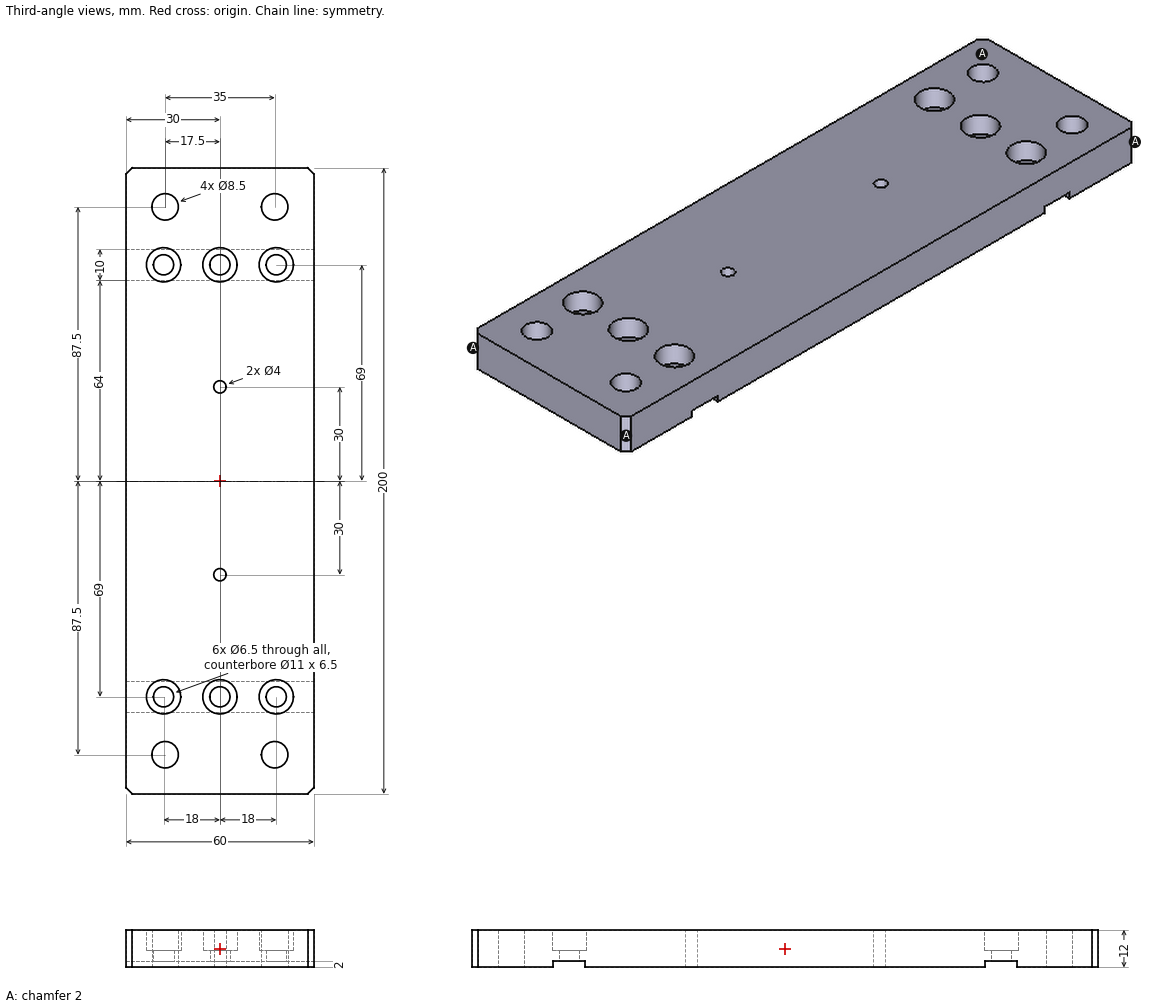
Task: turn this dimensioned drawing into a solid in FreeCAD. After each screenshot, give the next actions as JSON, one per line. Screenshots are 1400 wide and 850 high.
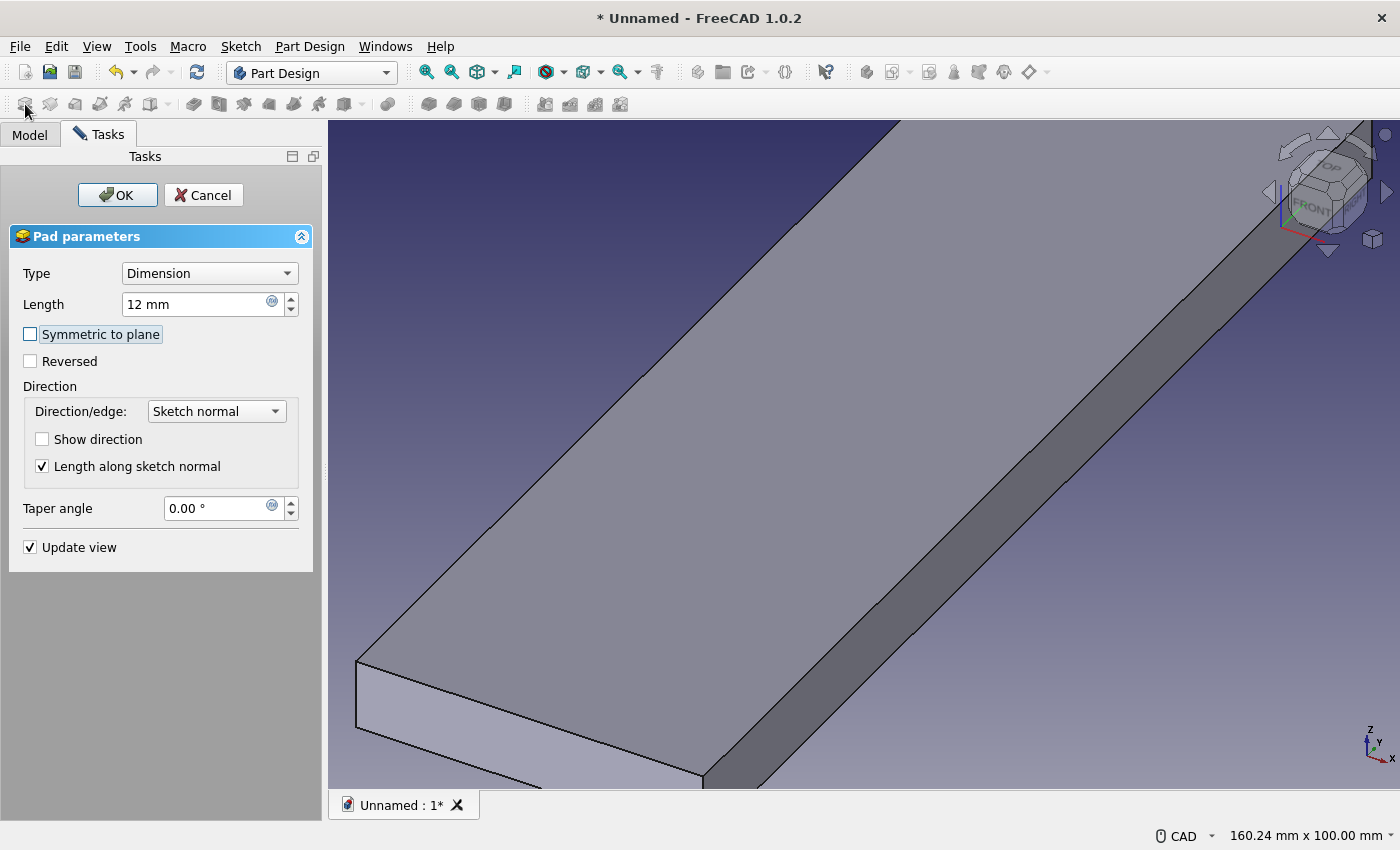
{"action": "left_click", "coordinate": [31, 334]}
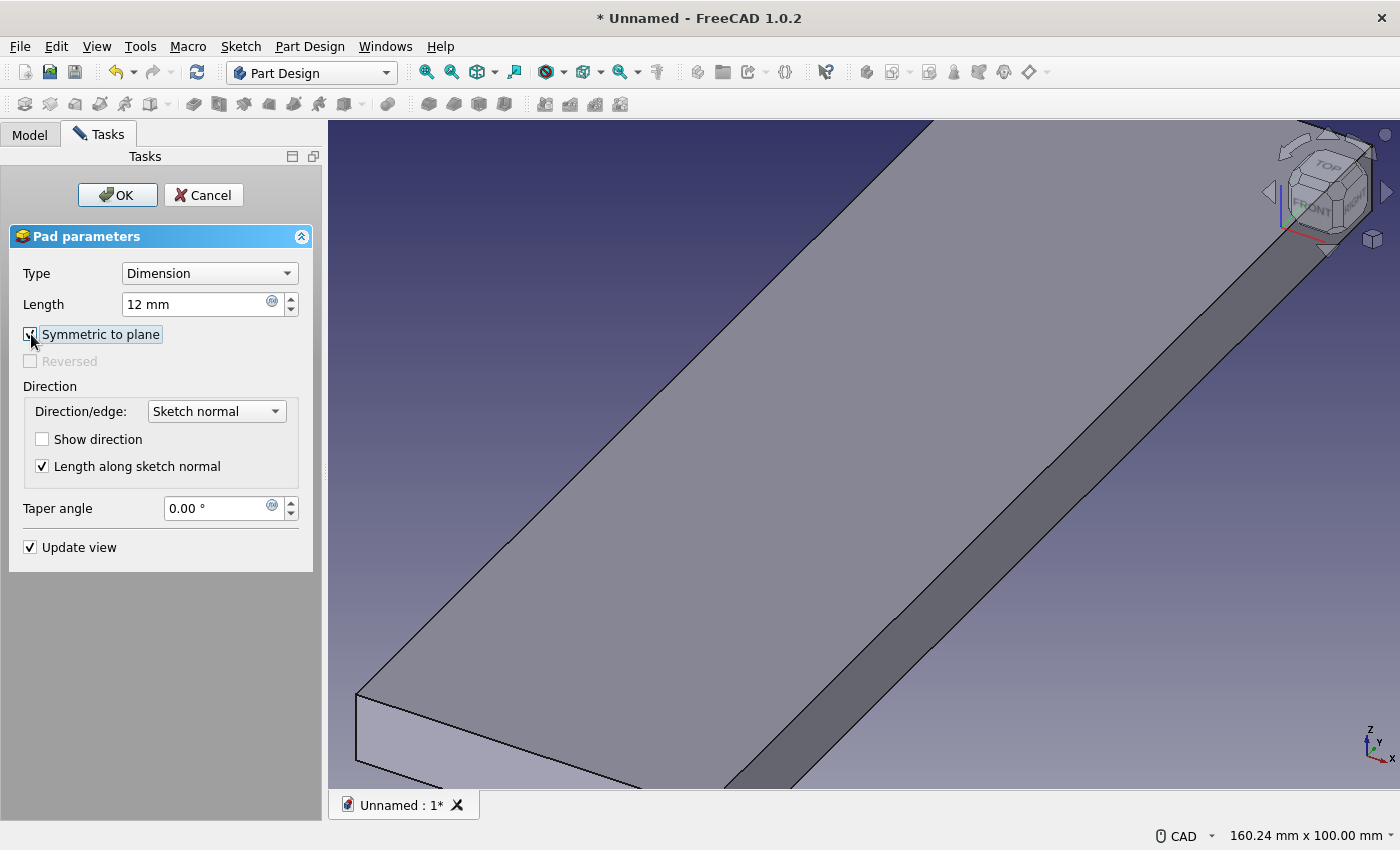
{"action": "left_click", "coordinate": [118, 195]}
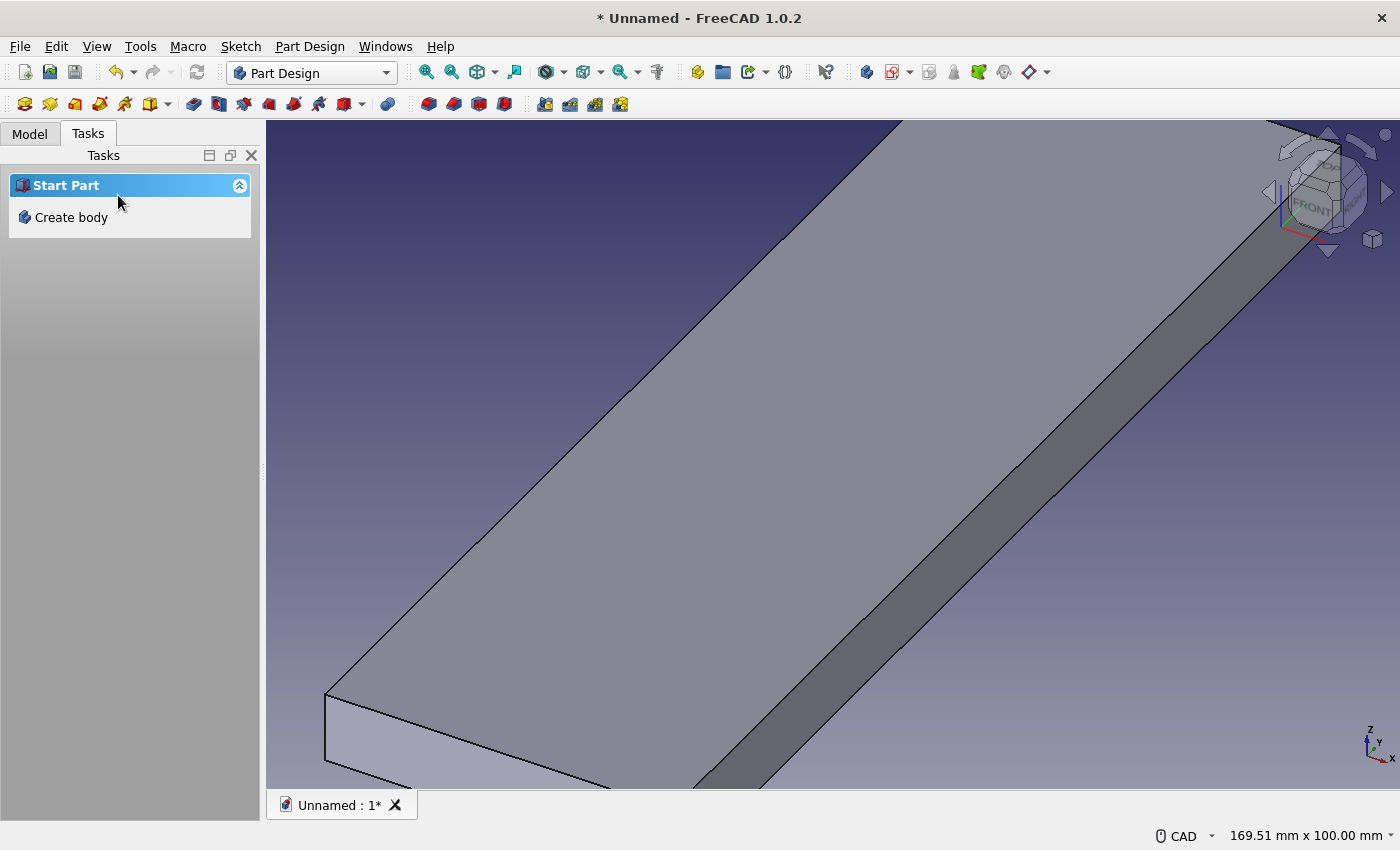
{"action": "left_click", "coordinate": [427, 72]}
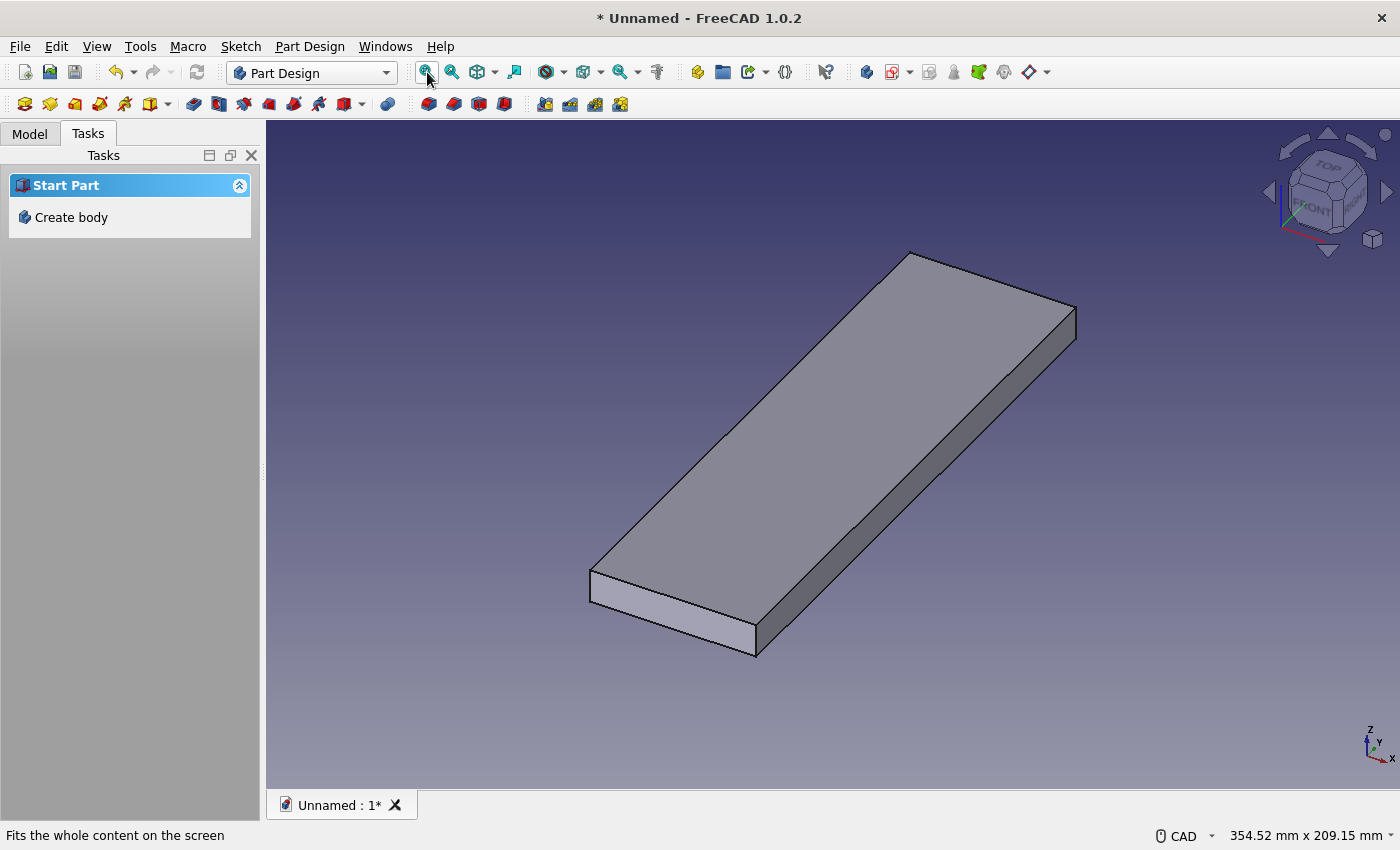
{"action": "left_click", "coordinate": [756, 640]}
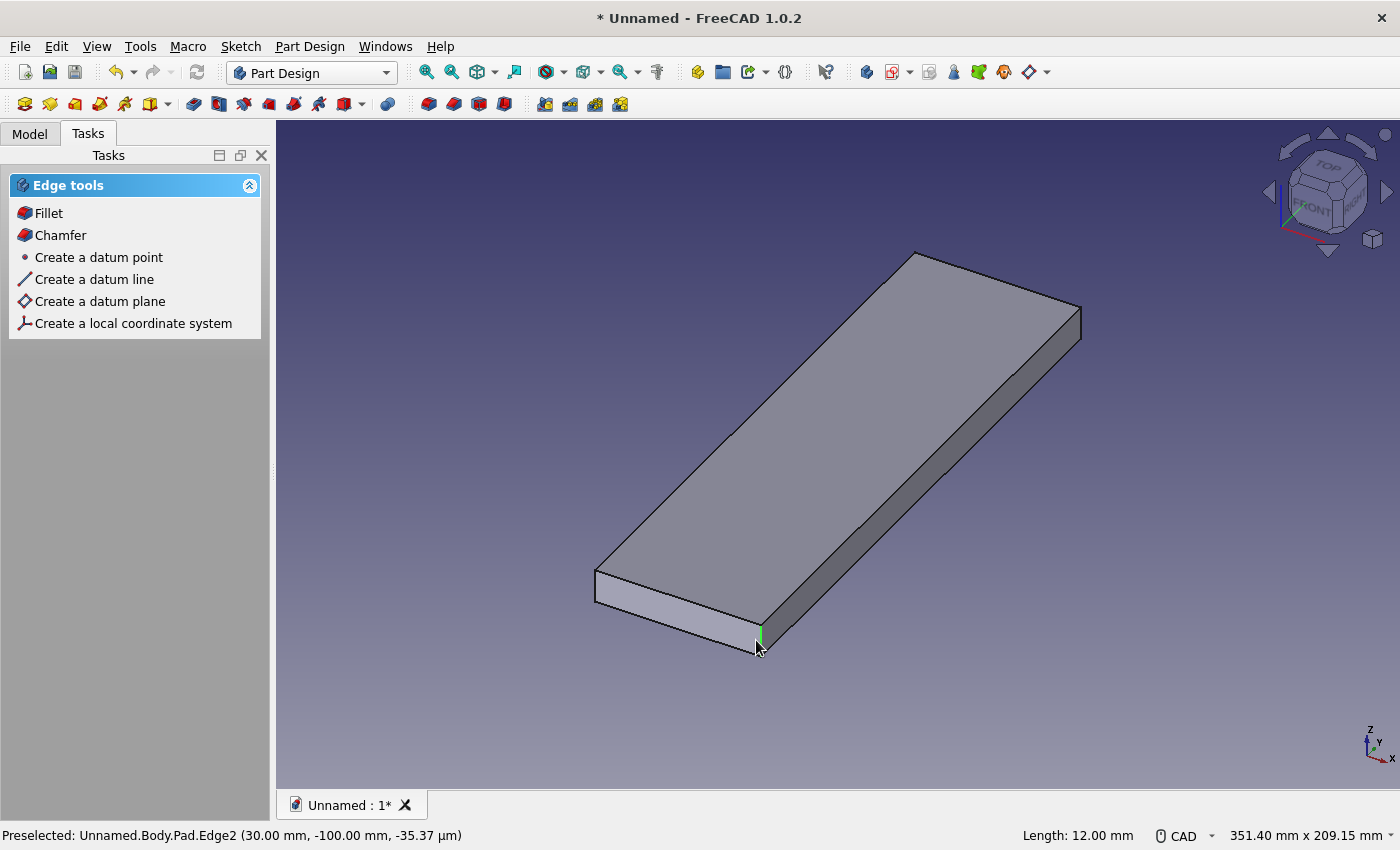
{"action": "key", "text": "0"}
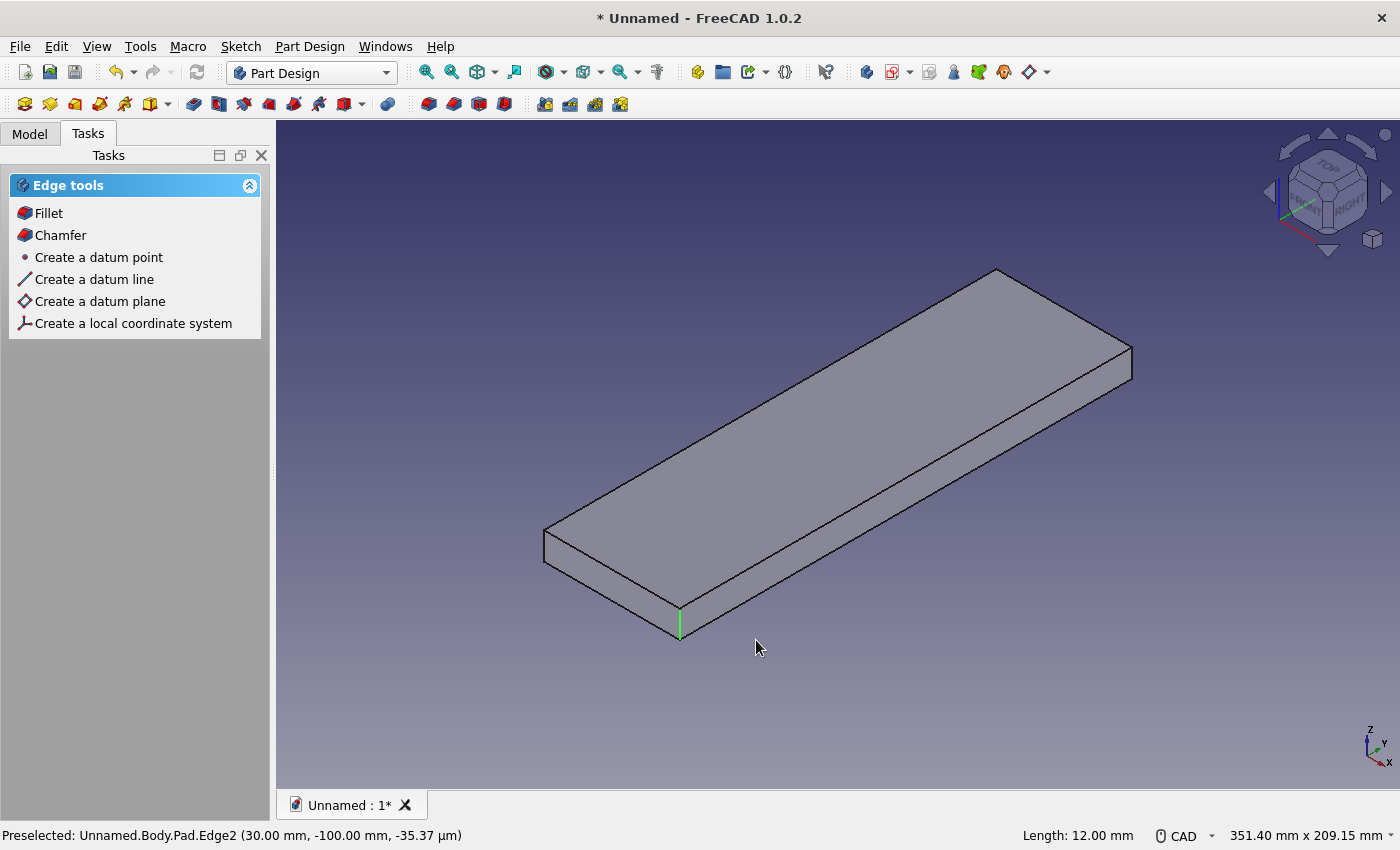
{"action": "key", "text": "2"}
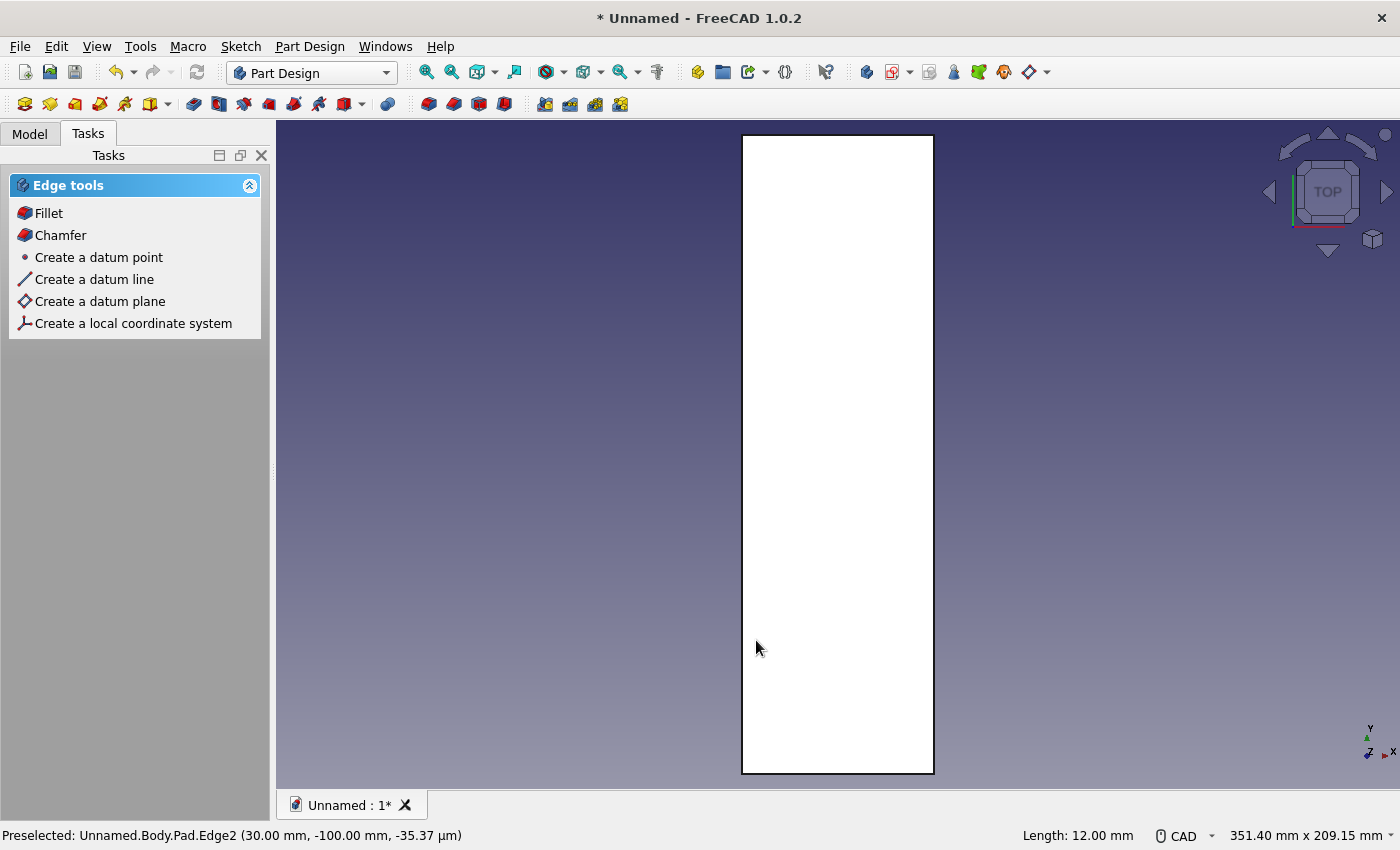
{"action": "key", "text": "1"}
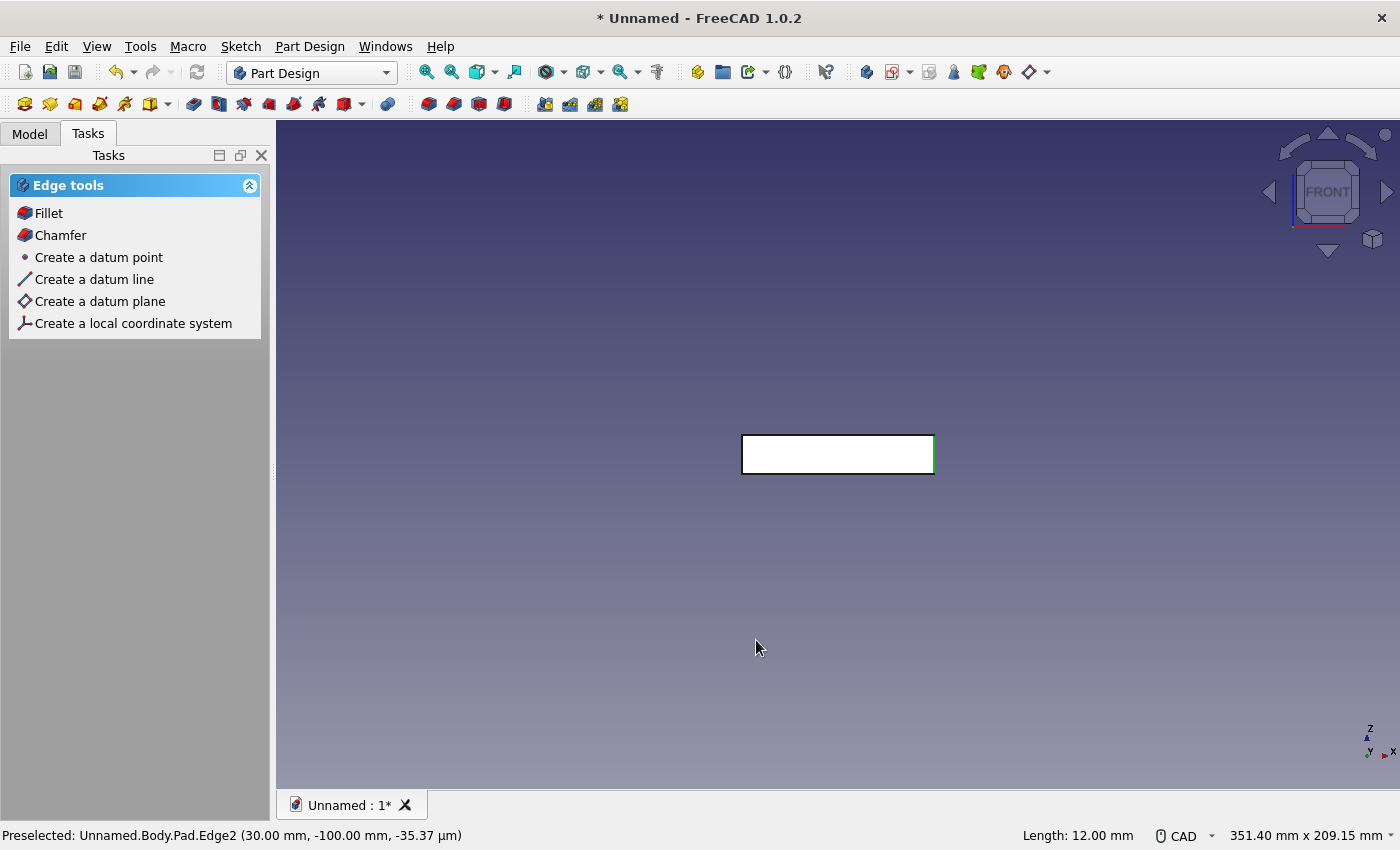
{"action": "left_click", "coordinate": [427, 72]}